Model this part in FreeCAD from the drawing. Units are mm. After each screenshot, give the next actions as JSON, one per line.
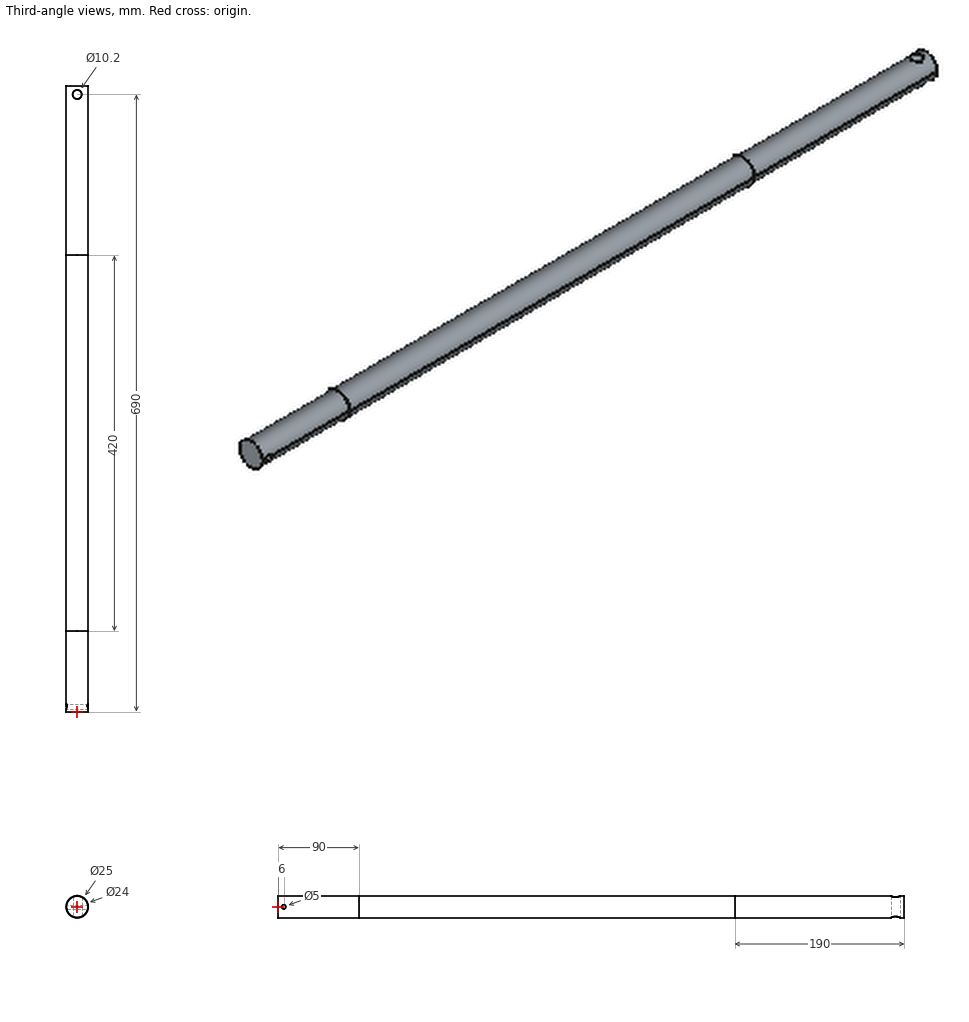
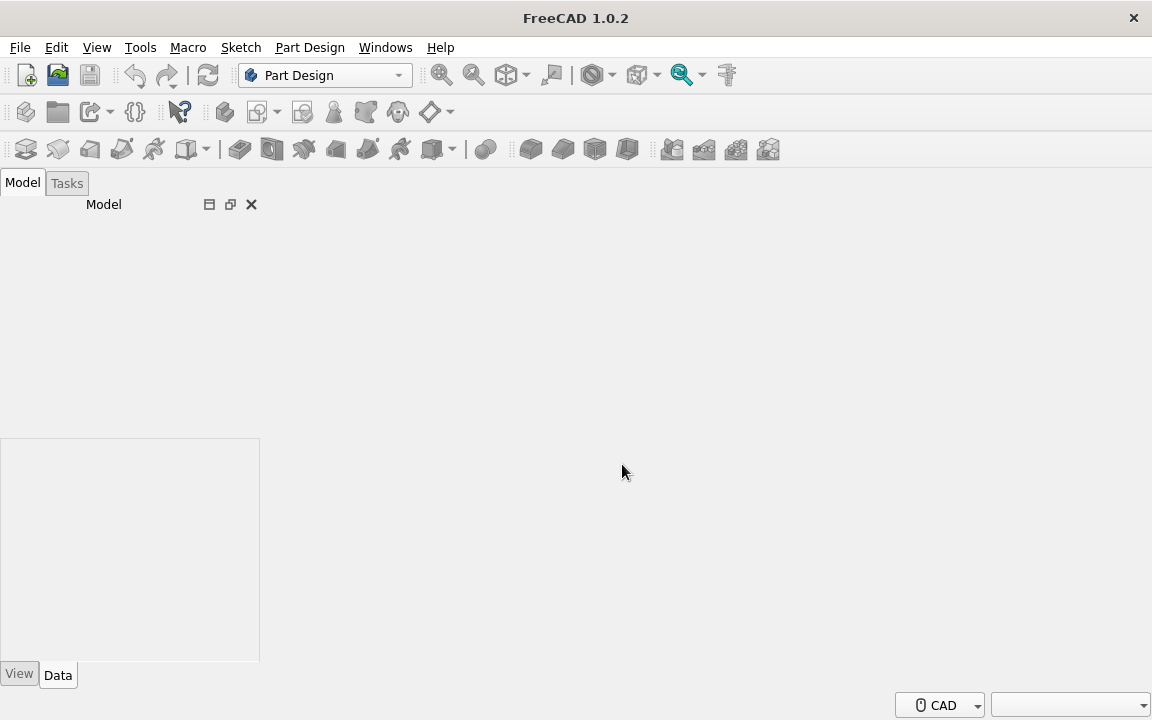
{"action": "left_click", "coordinate": [26, 76]}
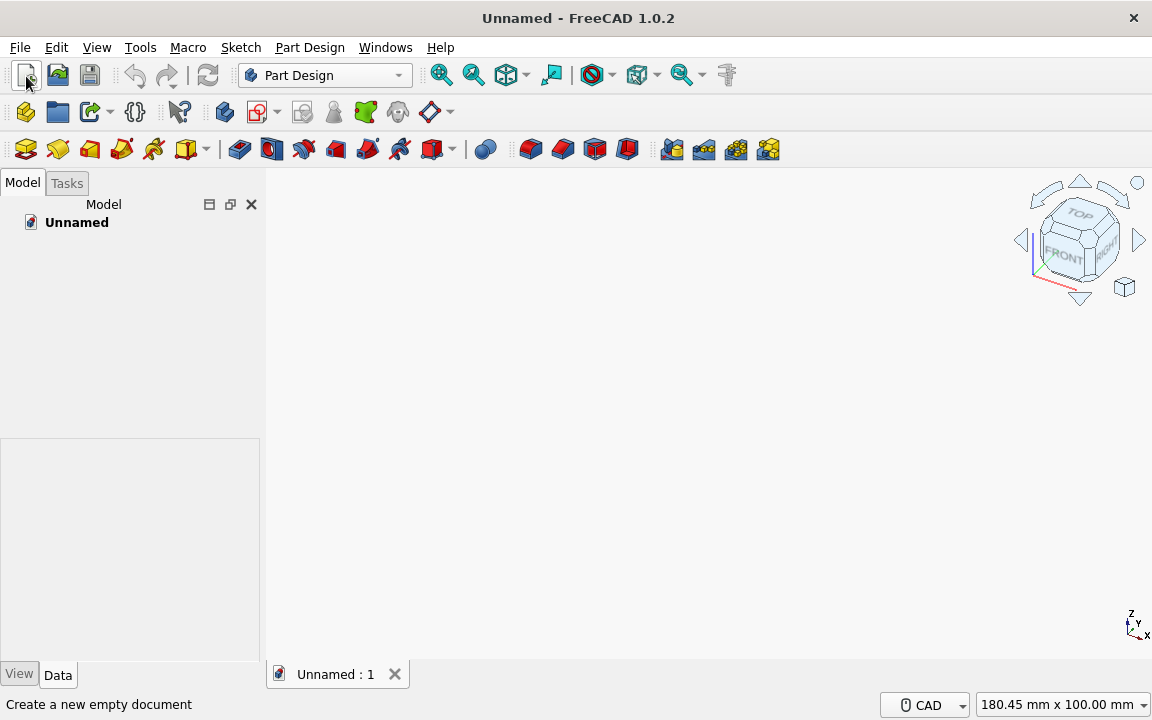
{"action": "left_click", "coordinate": [258, 112]}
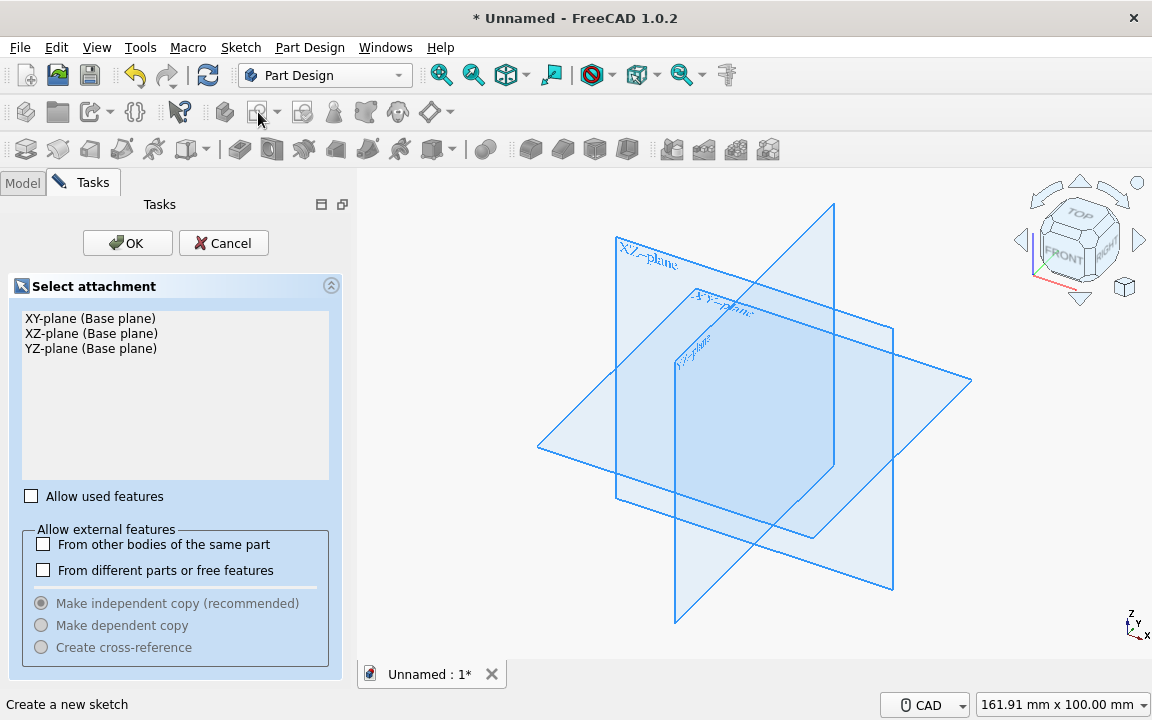
{"action": "left_click", "coordinate": [82, 334]}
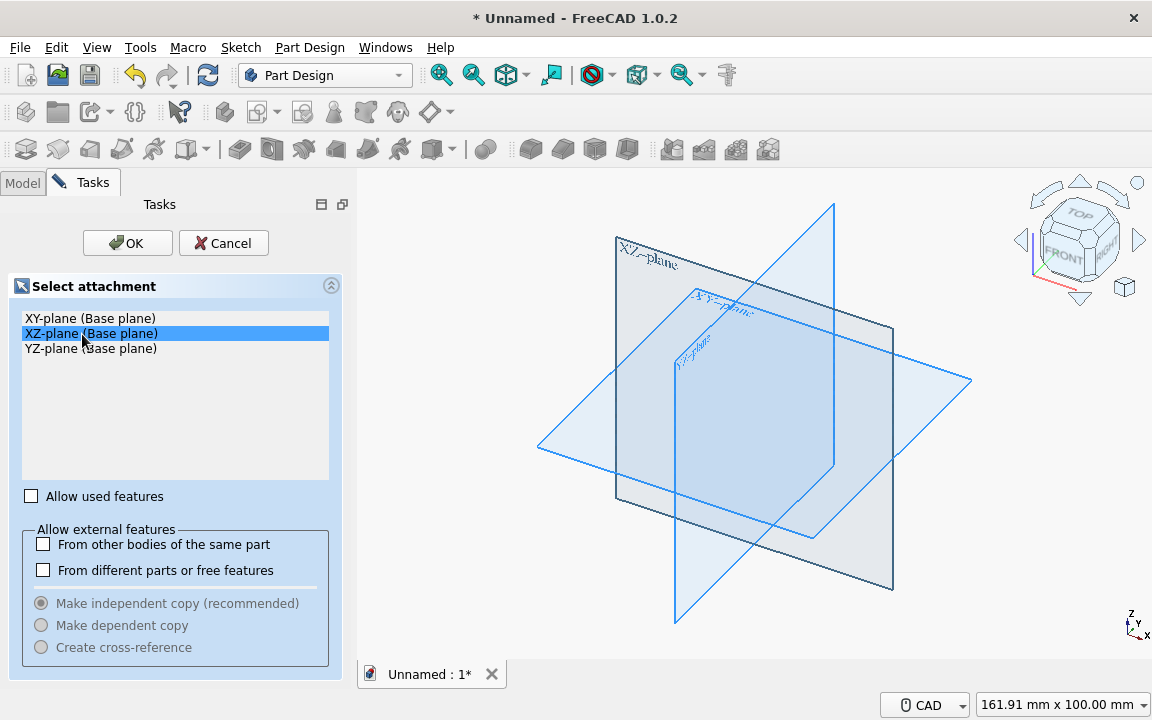
{"action": "left_click", "coordinate": [128, 243]}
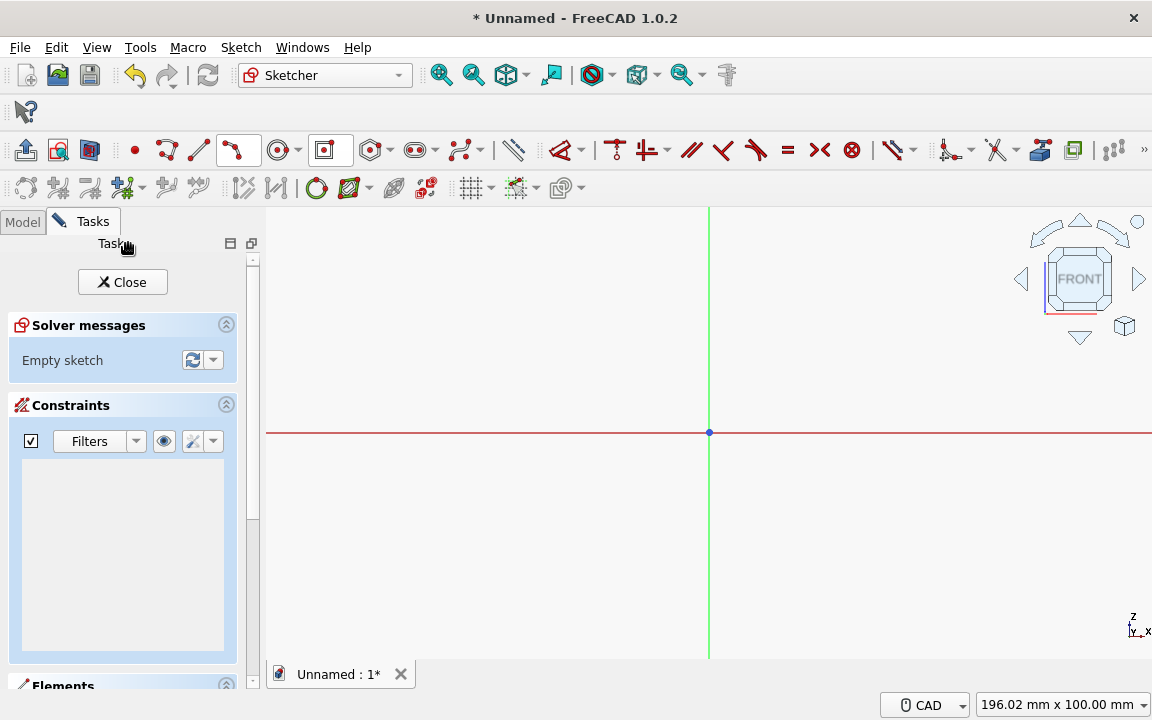
{"action": "scroll", "coordinate": [749, 433], "scroll_direction": "up", "scroll_amount": 5}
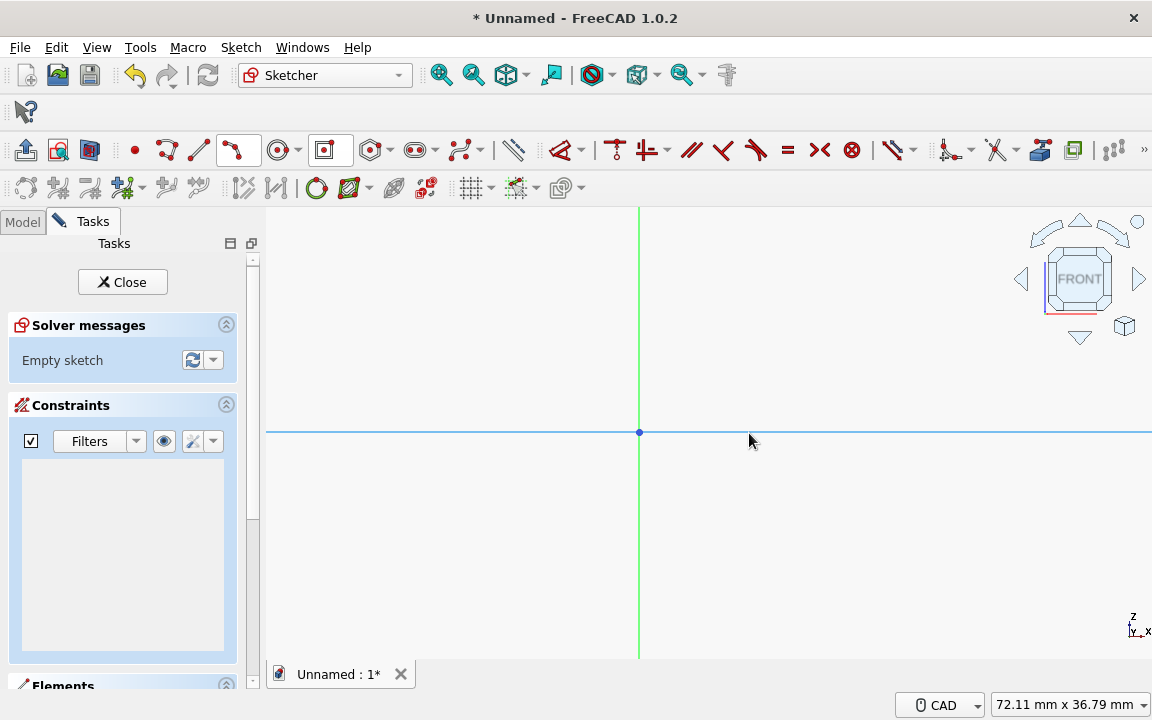
{"action": "left_click", "coordinate": [278, 150]}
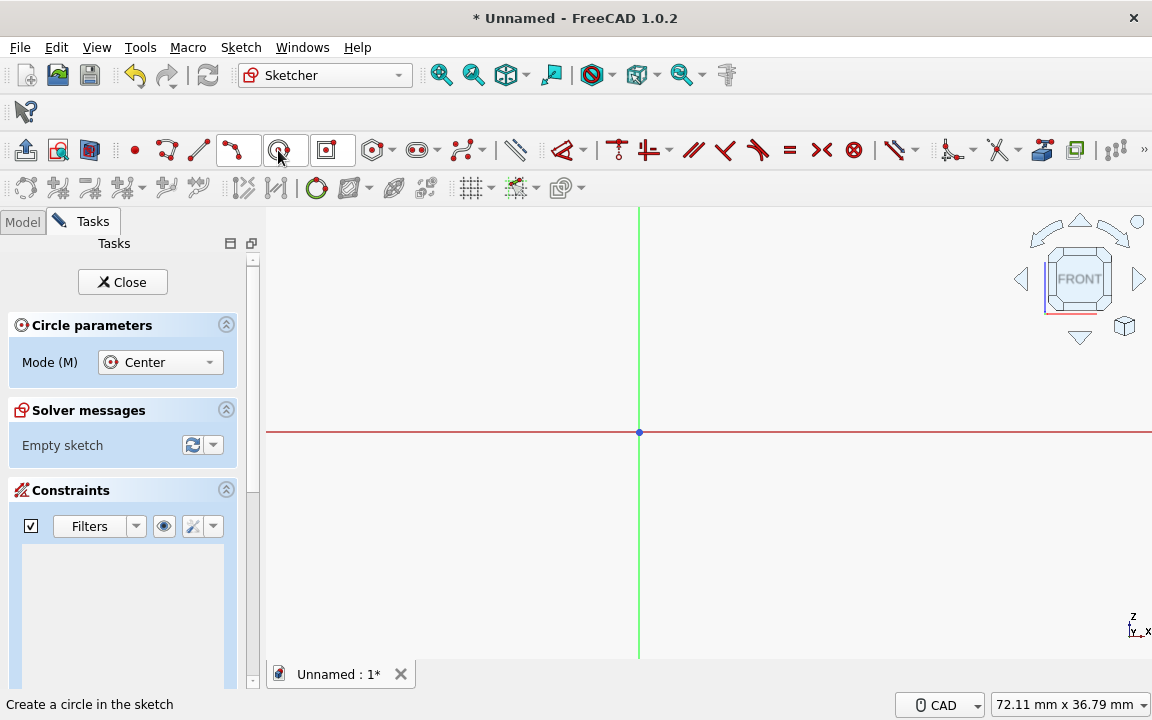
{"action": "left_click", "coordinate": [639, 432]}
{"action": "left_click", "coordinate": [744, 328]}
{"action": "key", "text": "Escape"}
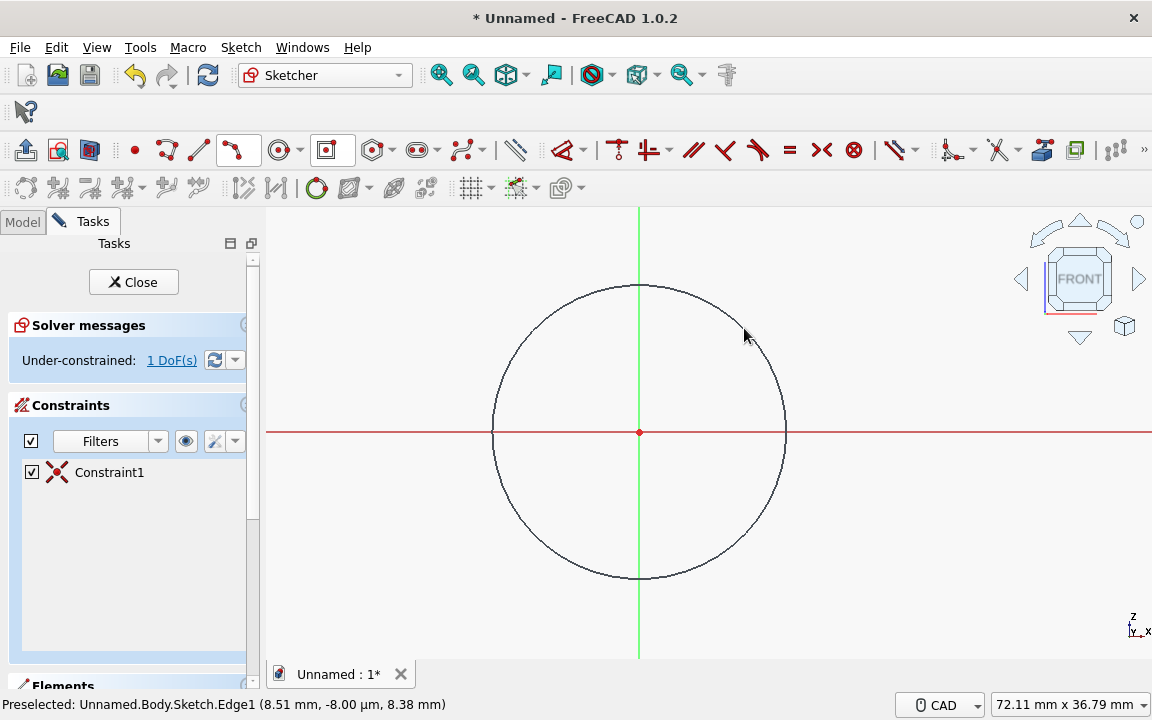
{"action": "left_click", "coordinate": [743, 328]}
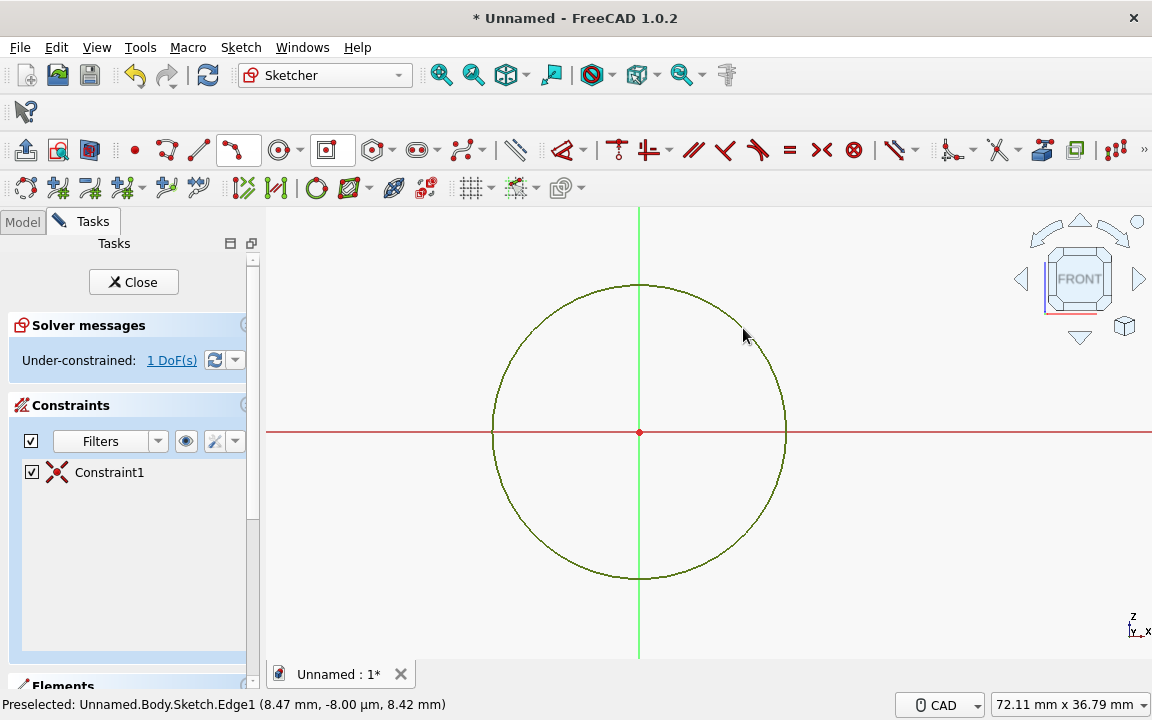
{"action": "key", "text": "k o"}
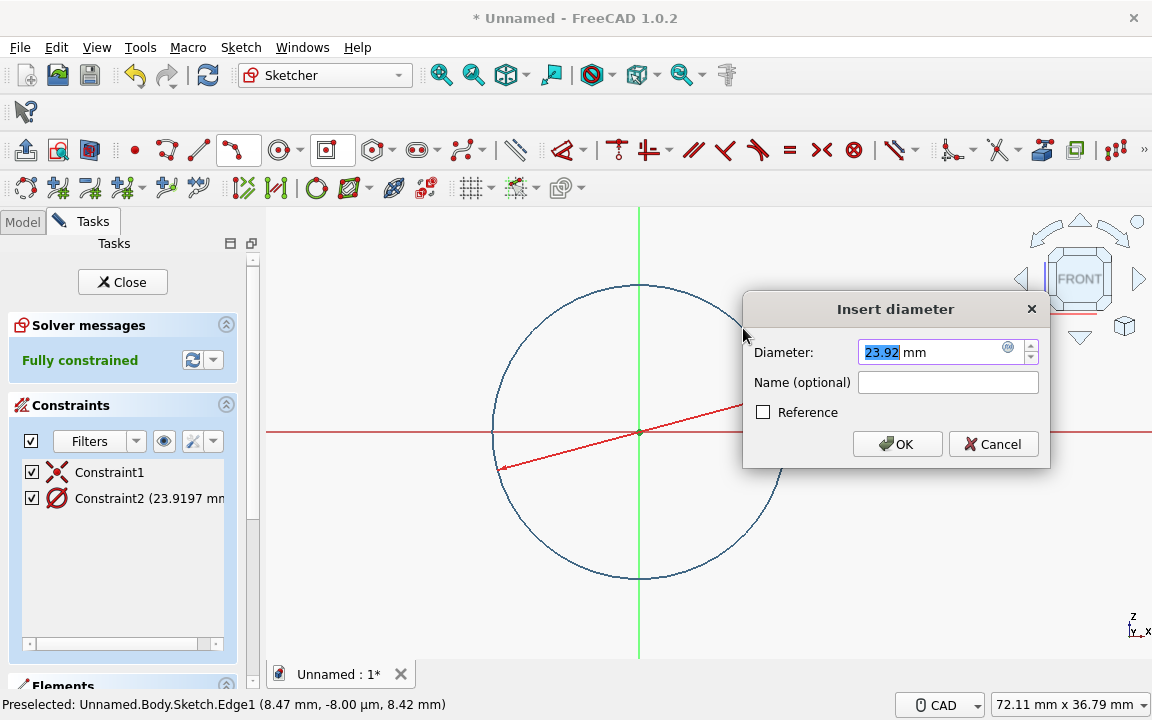
{"action": "type", "text": "24"}
{"action": "key", "text": "Return"}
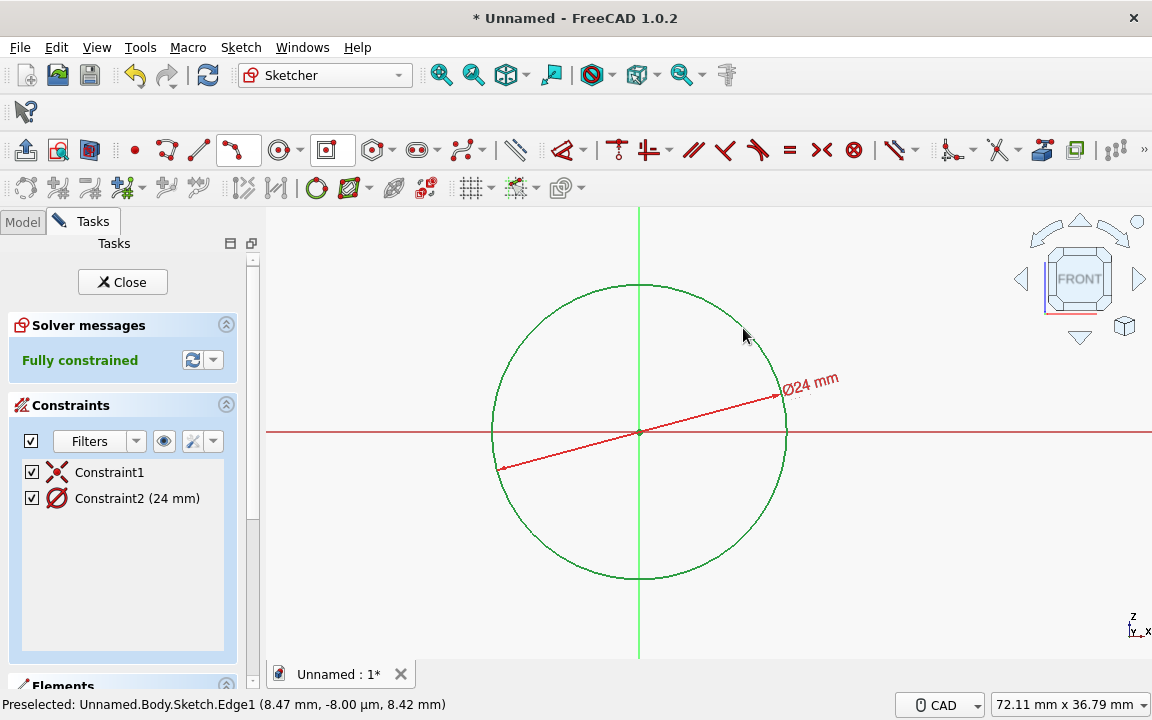
{"action": "left_click", "coordinate": [123, 282]}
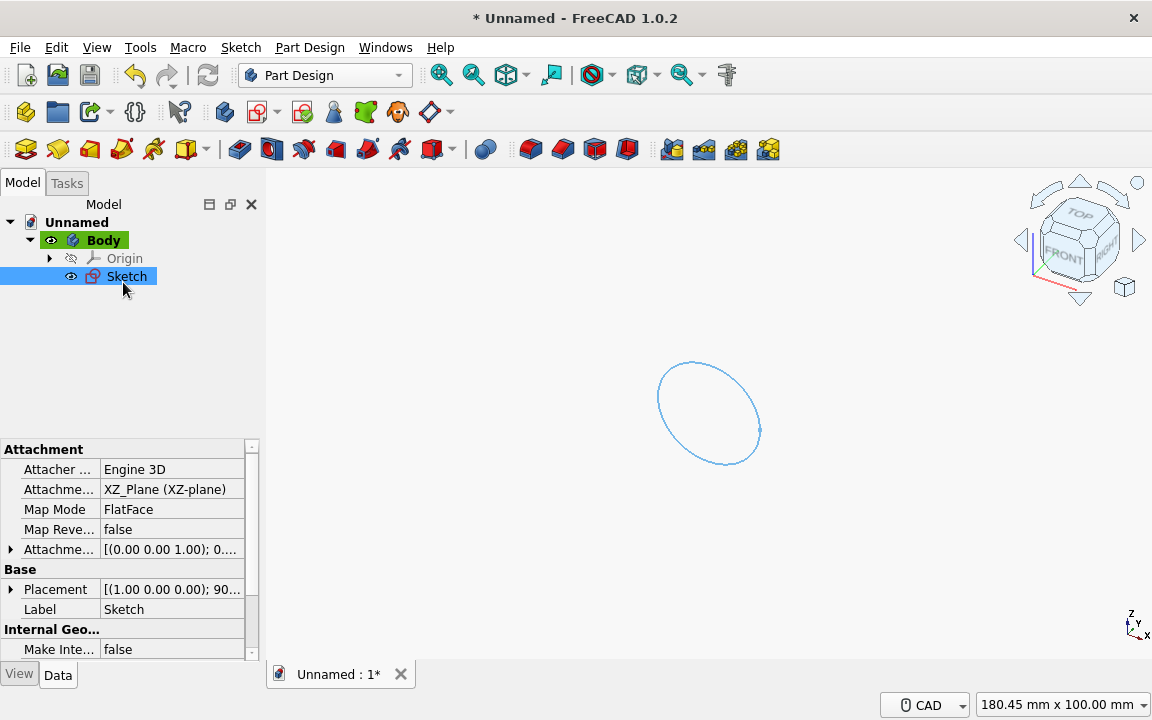
{"action": "left_click", "coordinate": [26, 150]}